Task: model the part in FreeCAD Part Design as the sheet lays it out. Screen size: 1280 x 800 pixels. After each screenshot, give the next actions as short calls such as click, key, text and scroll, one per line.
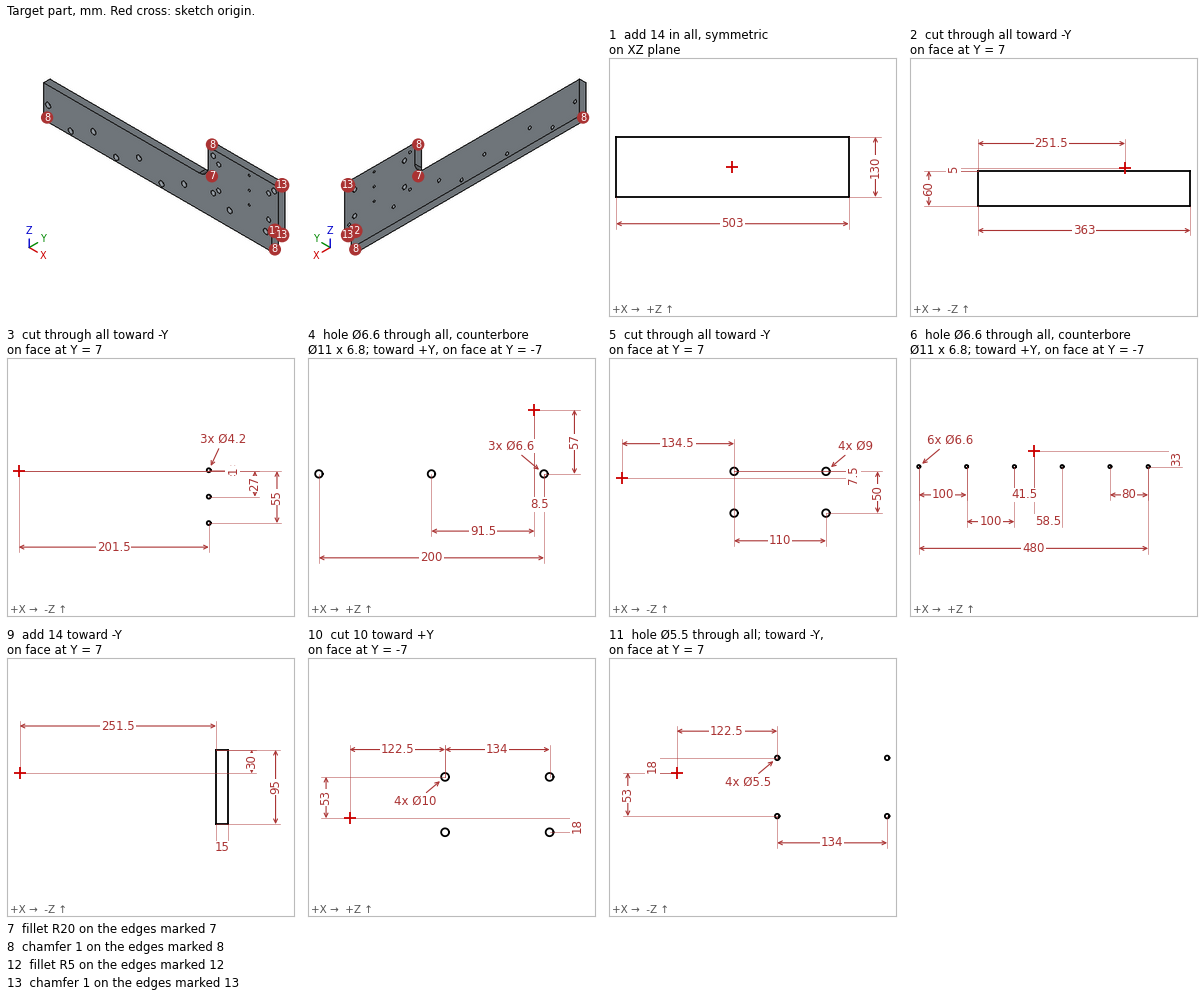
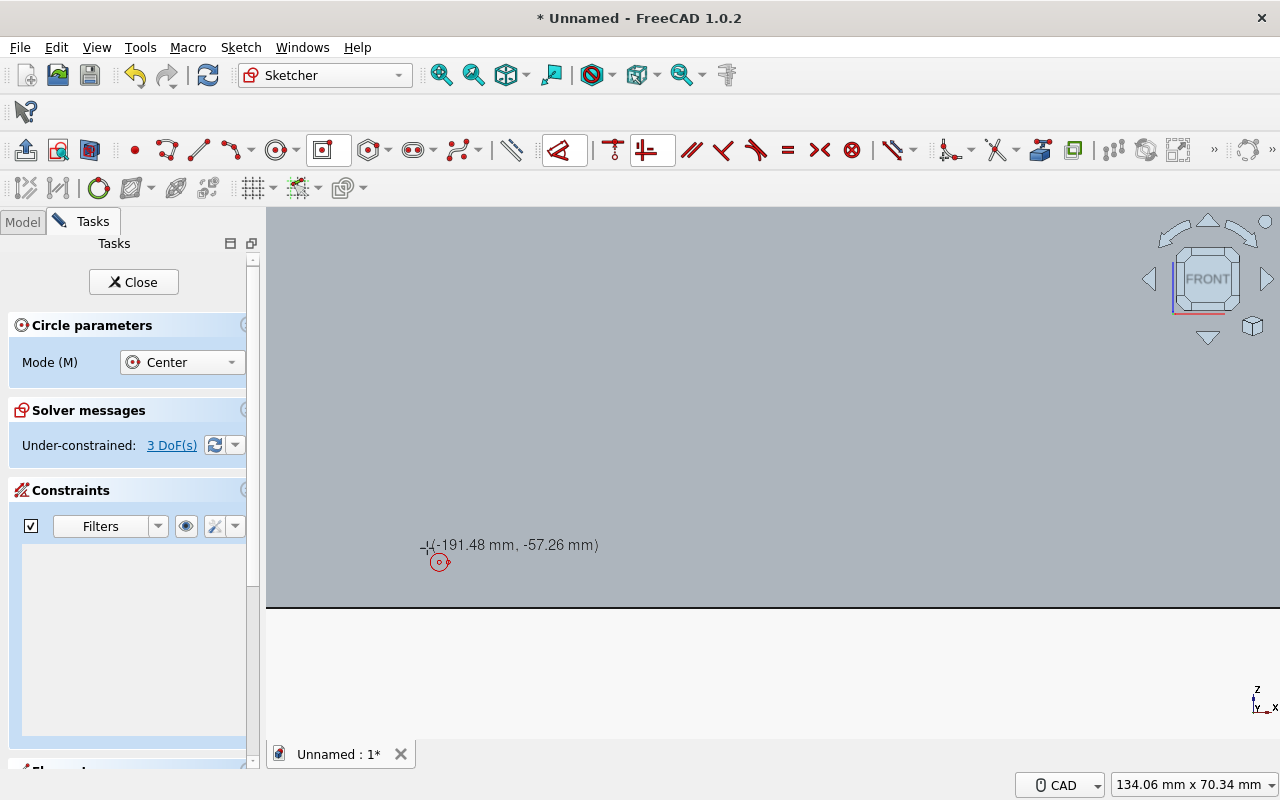
click(427, 548)
click(444, 530)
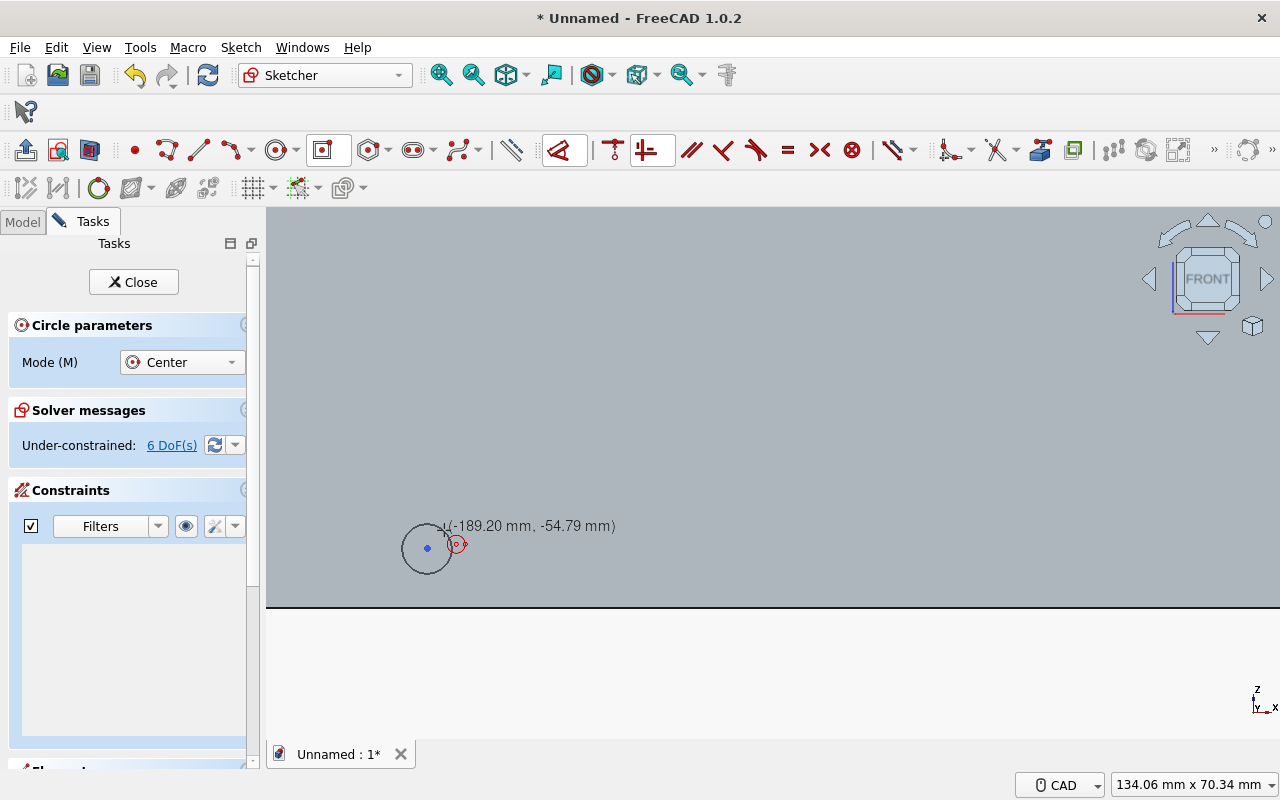
scroll(426, 548, down, 5)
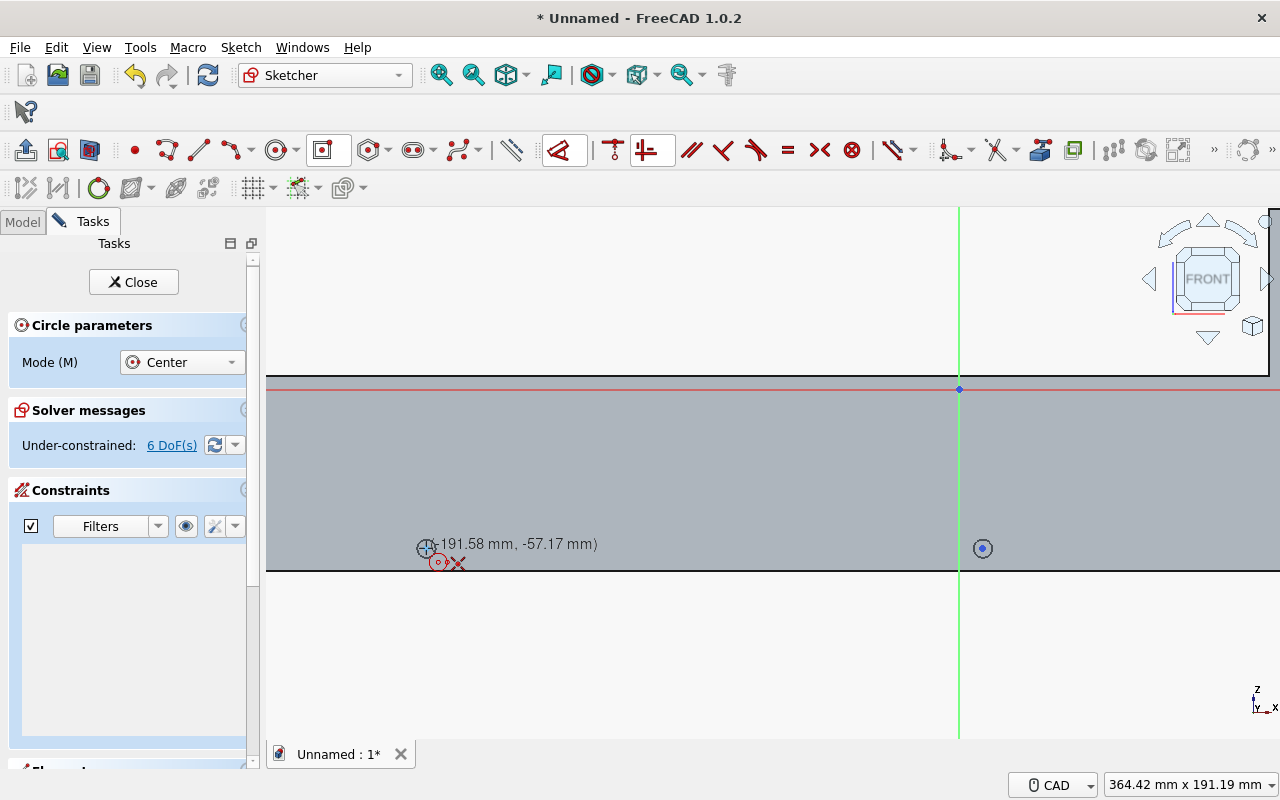
scroll(705, 548, up, 5)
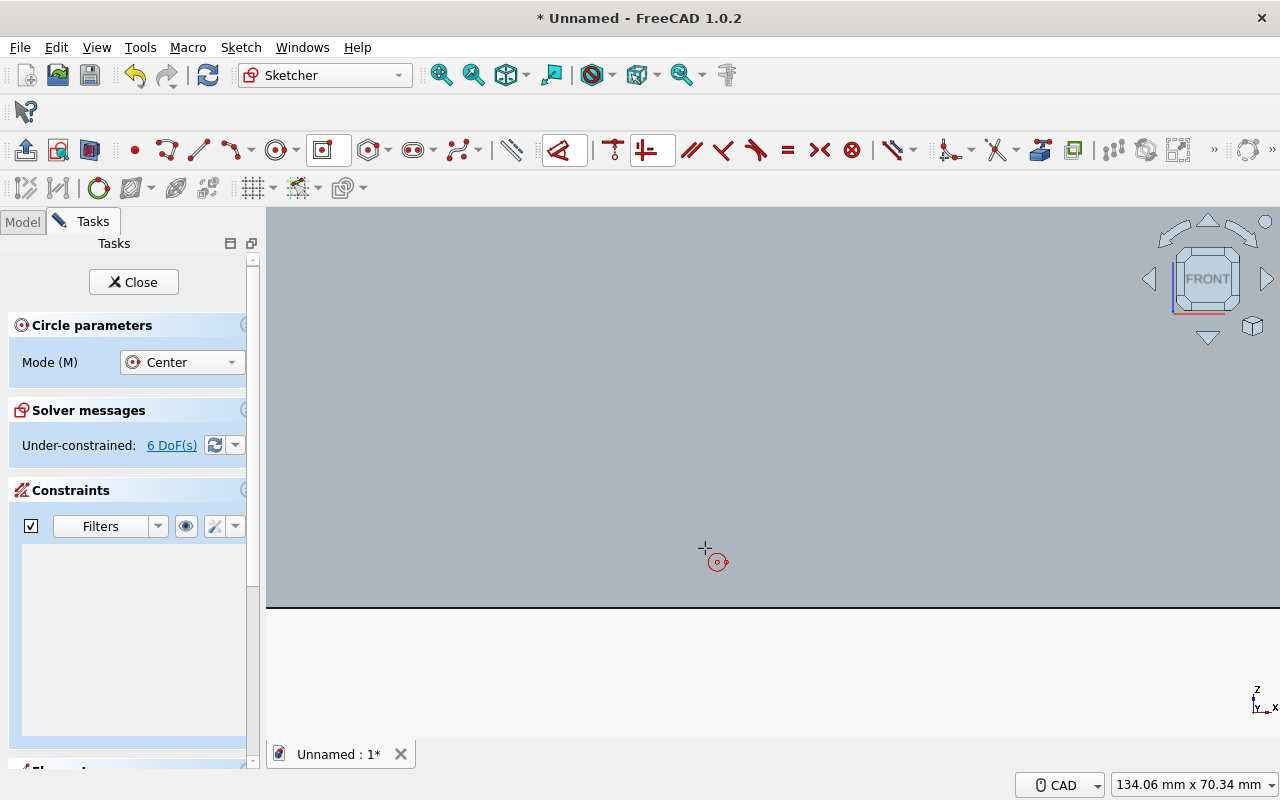
click(703, 548)
click(721, 530)
key(Escape)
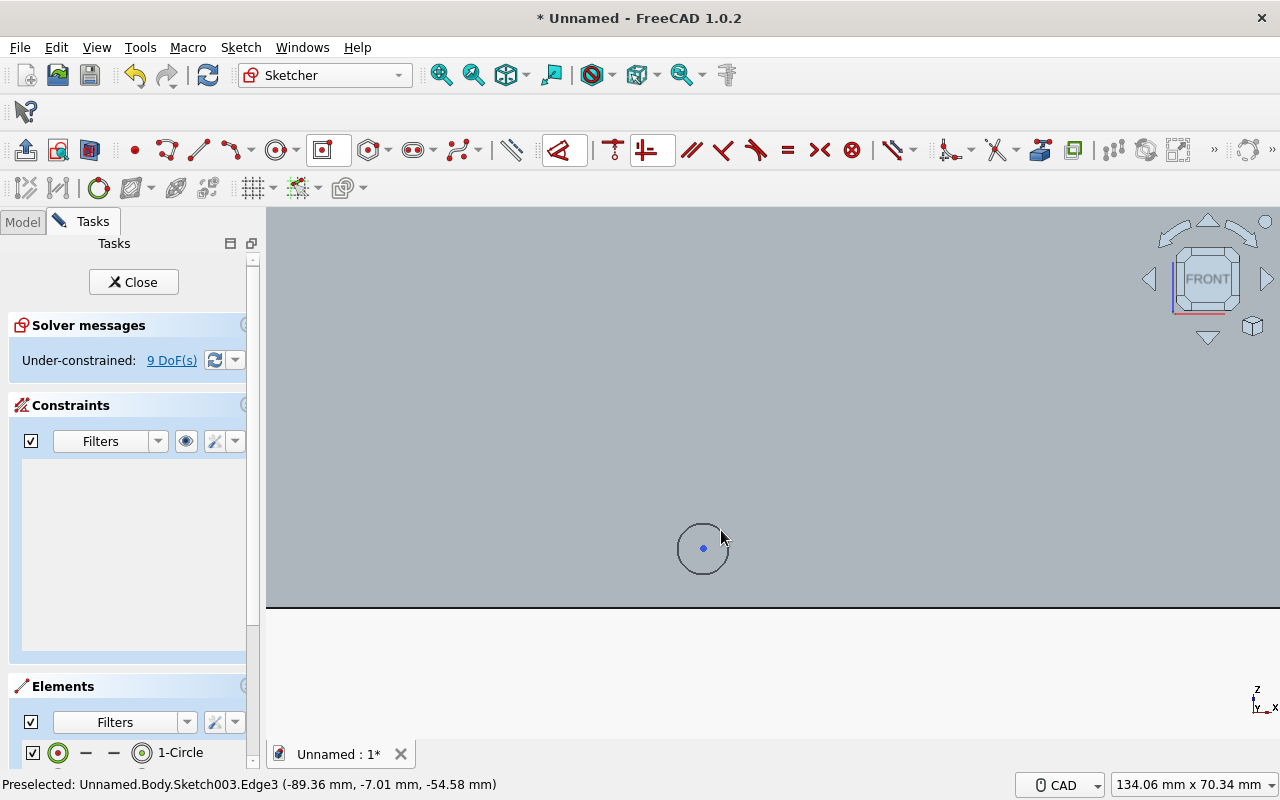
scroll(705, 548, down, 5)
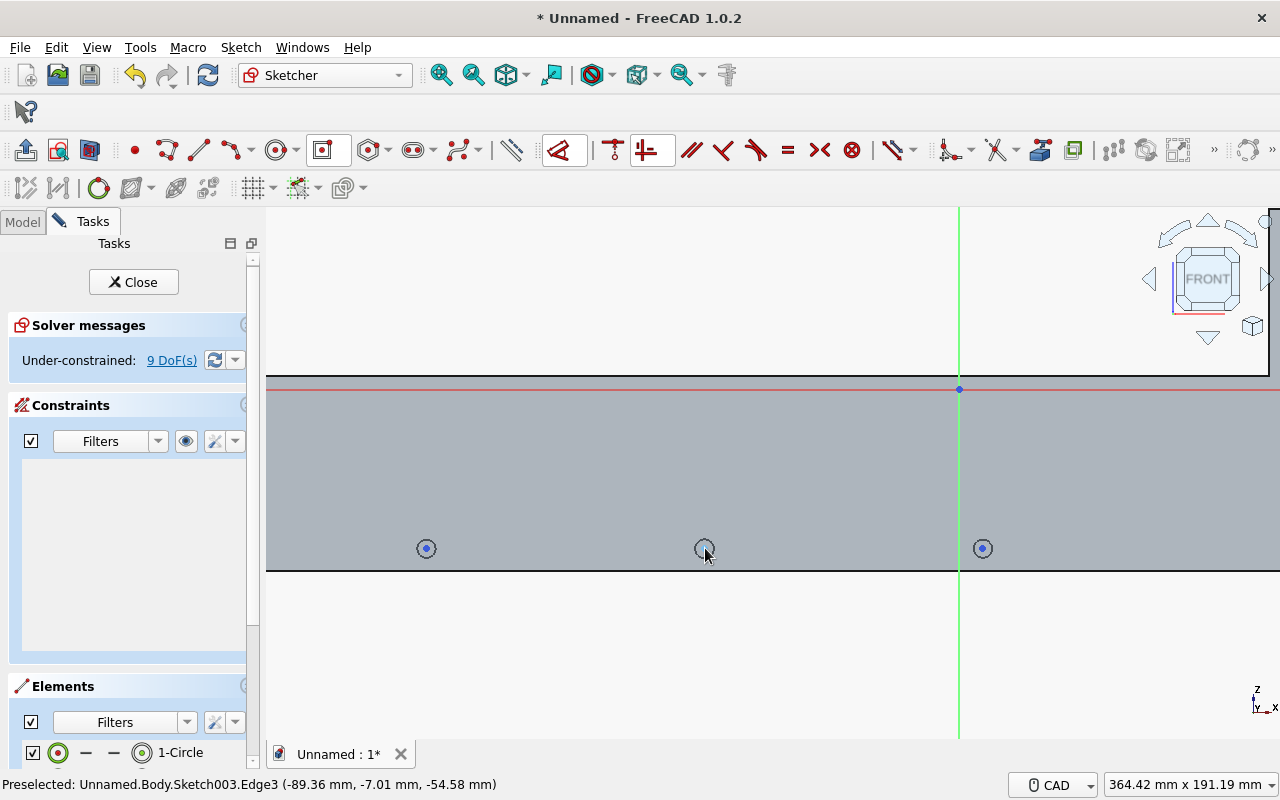
scroll(989, 542, up, 3)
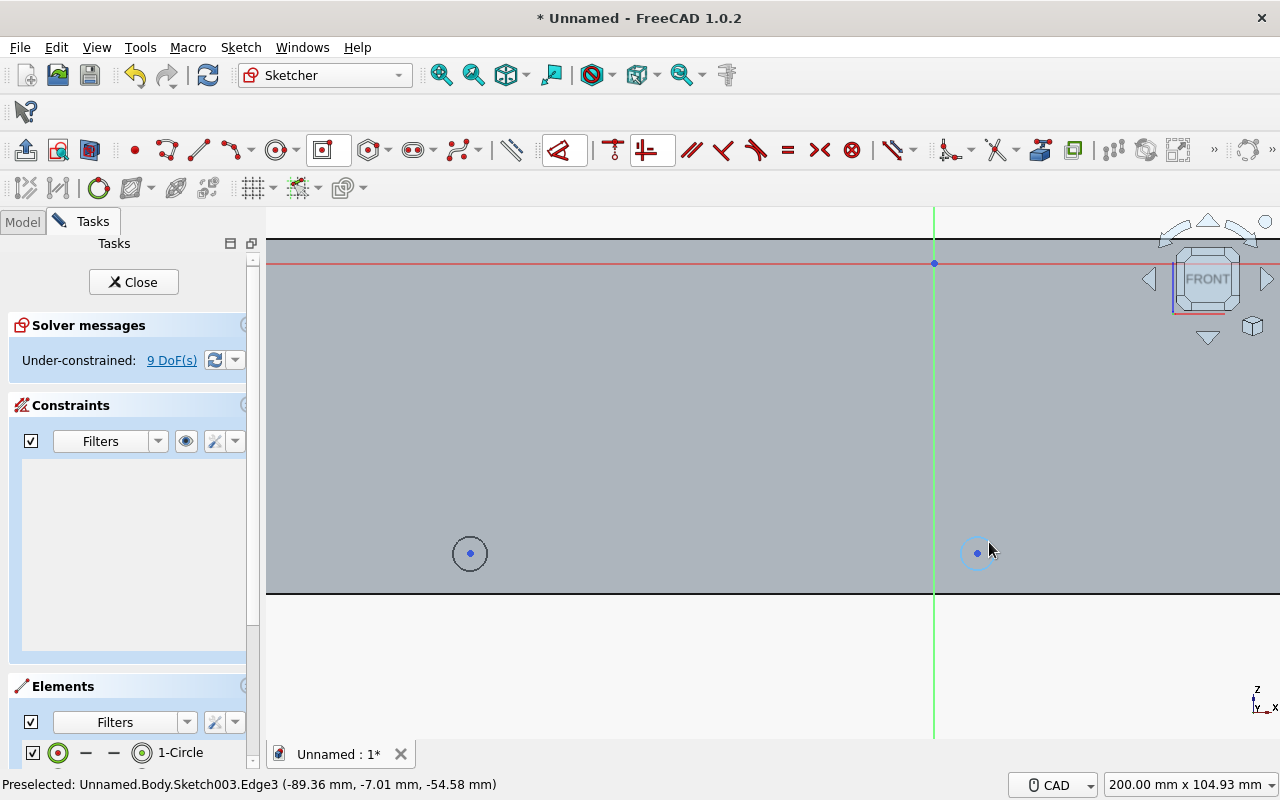
click(989, 542)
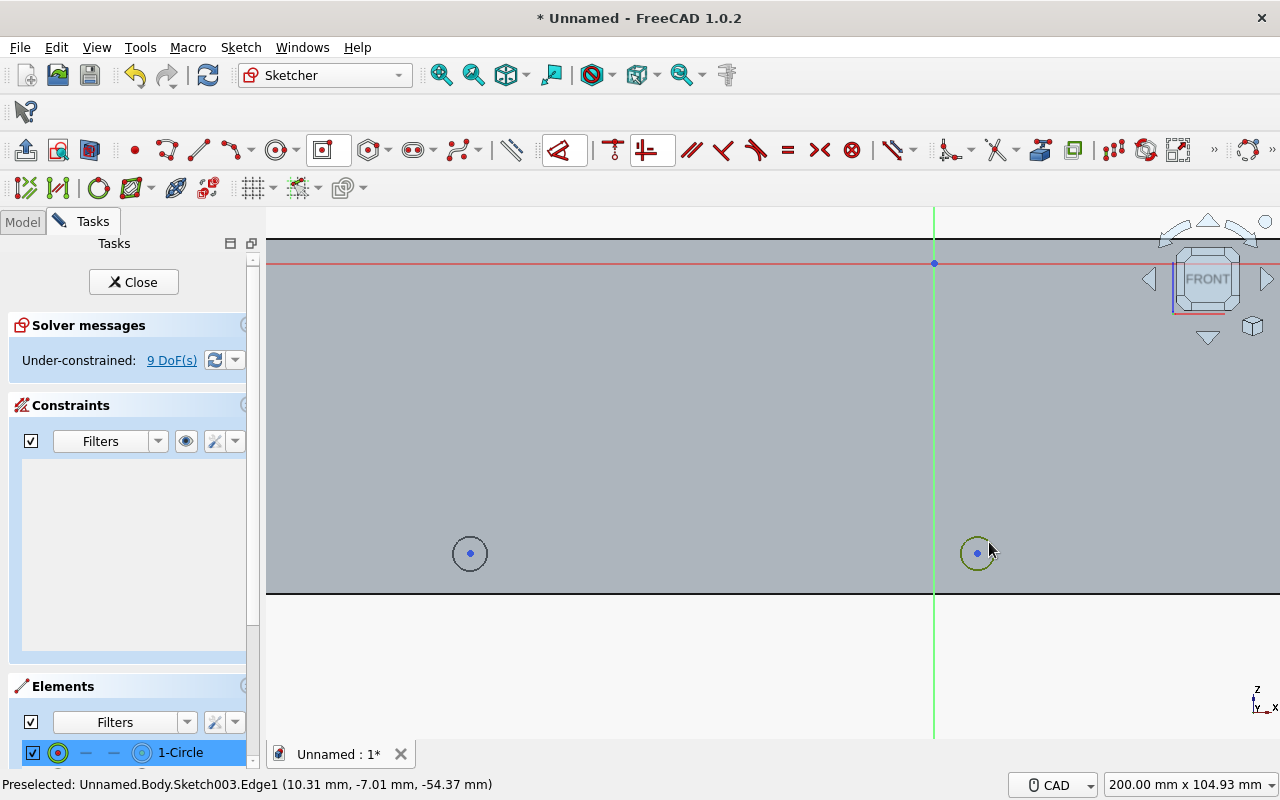
scroll(990, 541, down, 3)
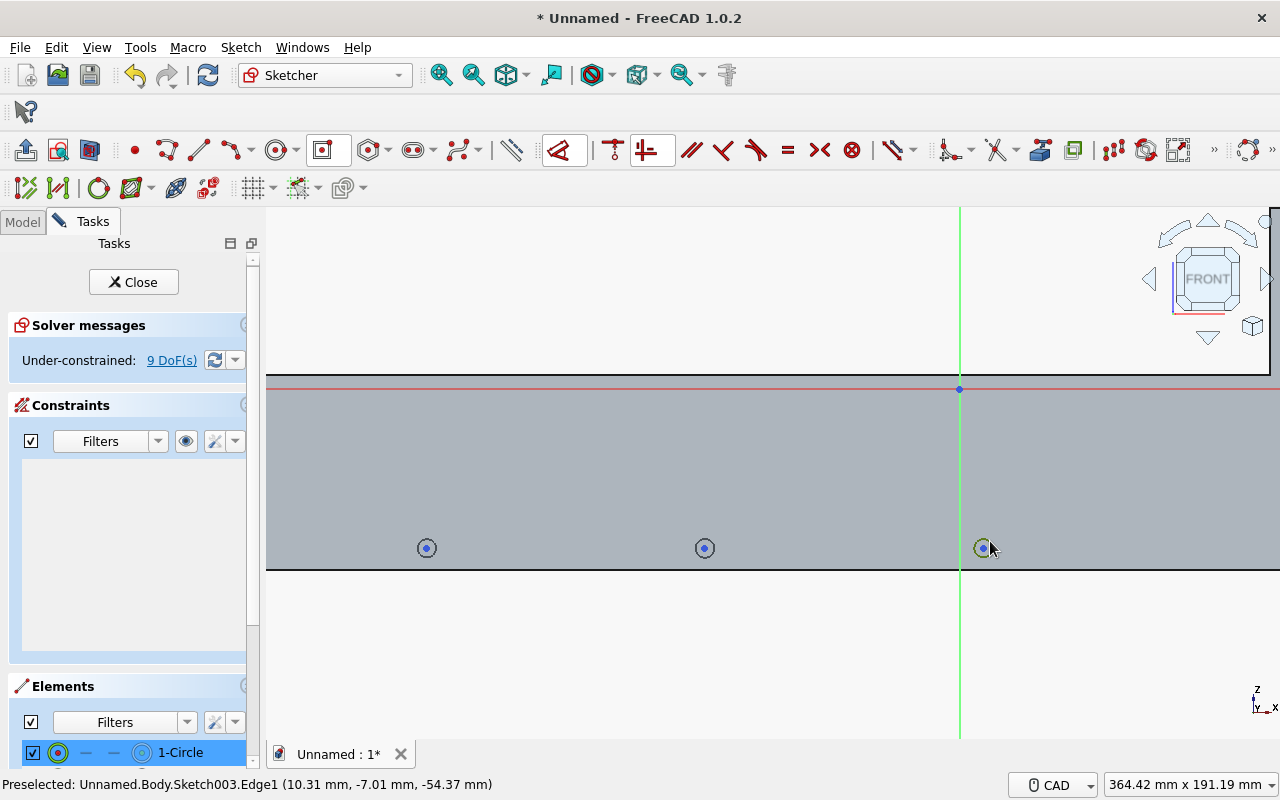
scroll(433, 542, up, 3)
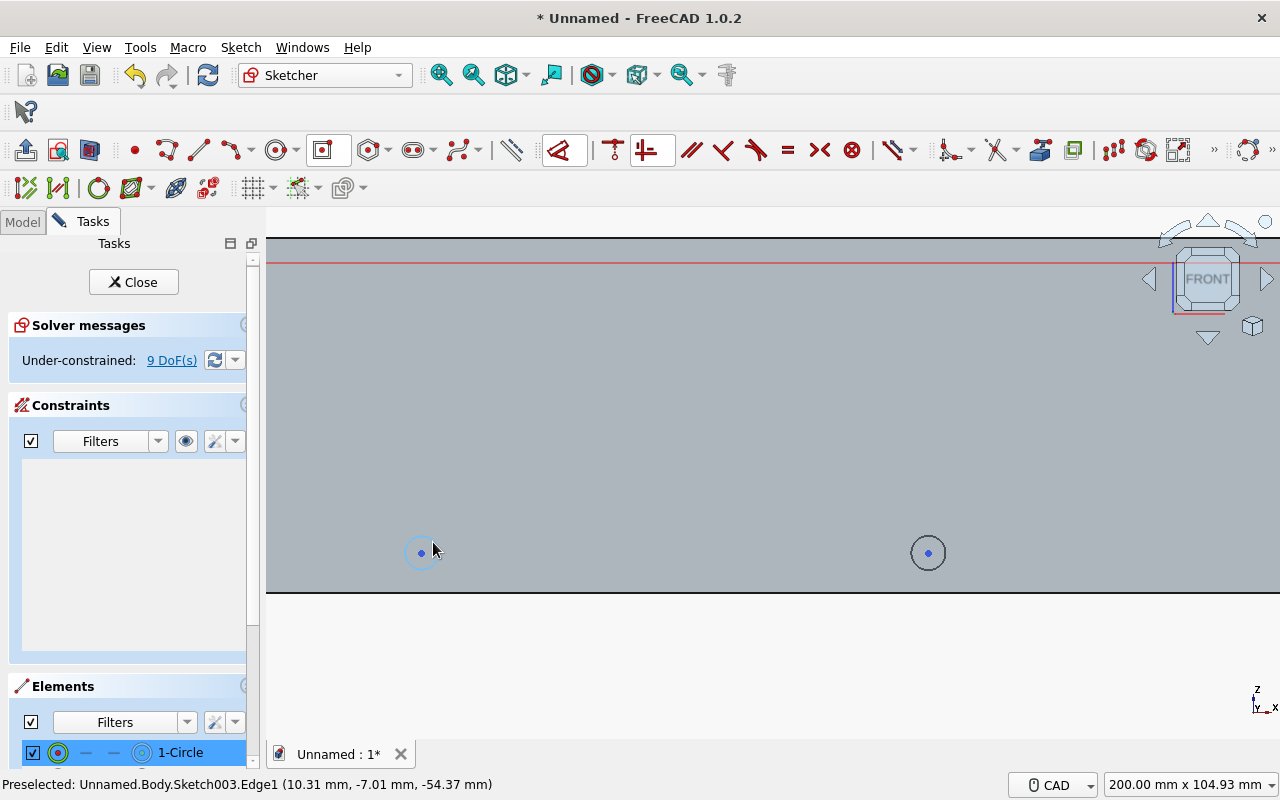
click(433, 541)